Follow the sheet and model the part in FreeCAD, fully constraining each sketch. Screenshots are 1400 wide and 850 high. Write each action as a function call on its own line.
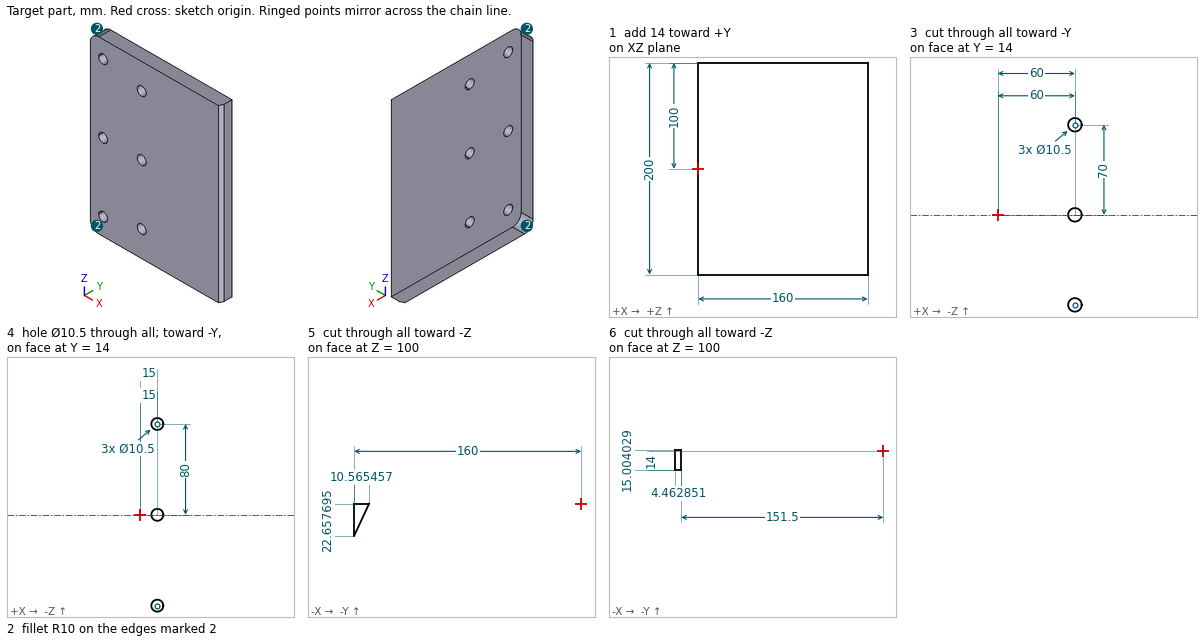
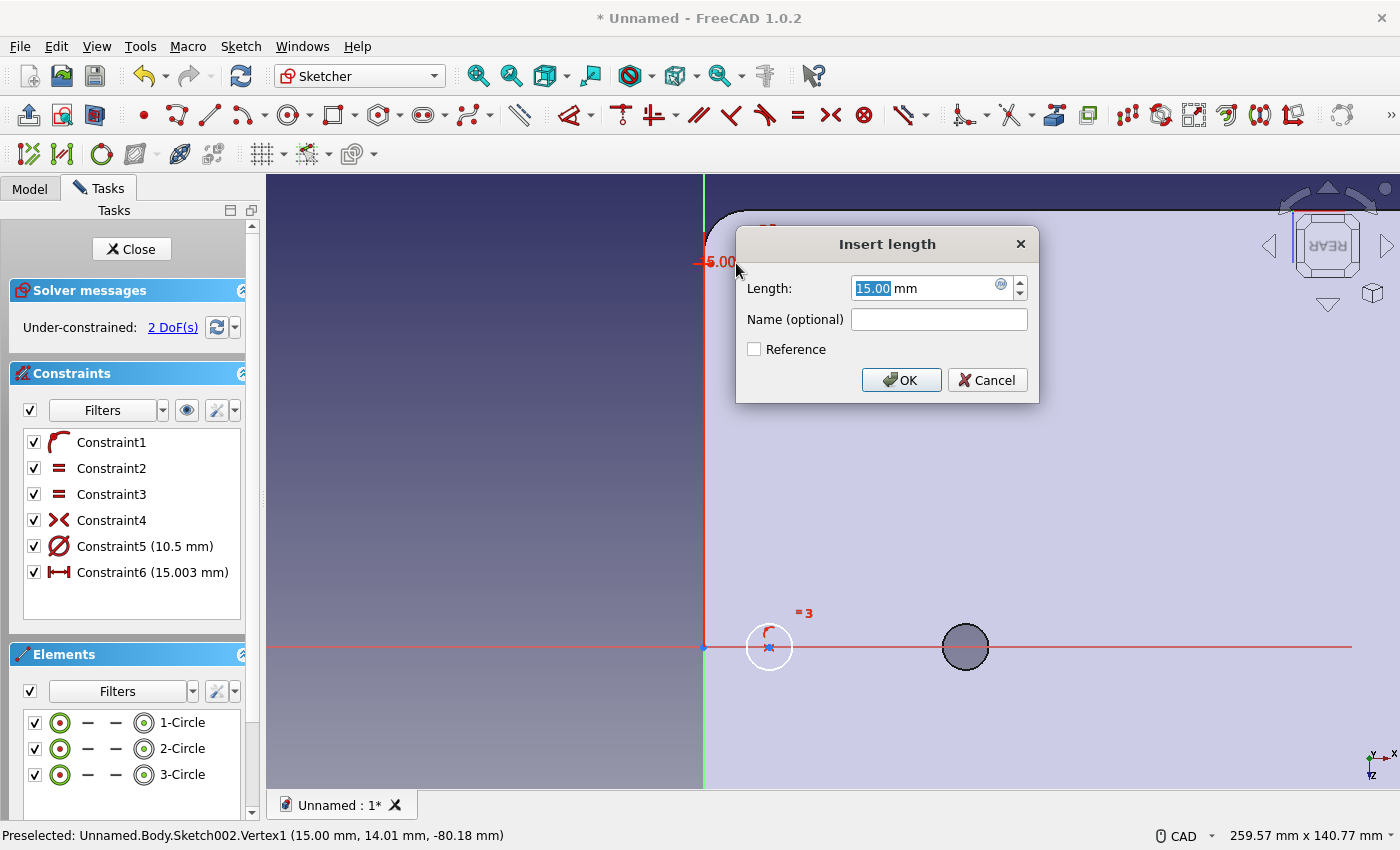
text(15)
key(Return)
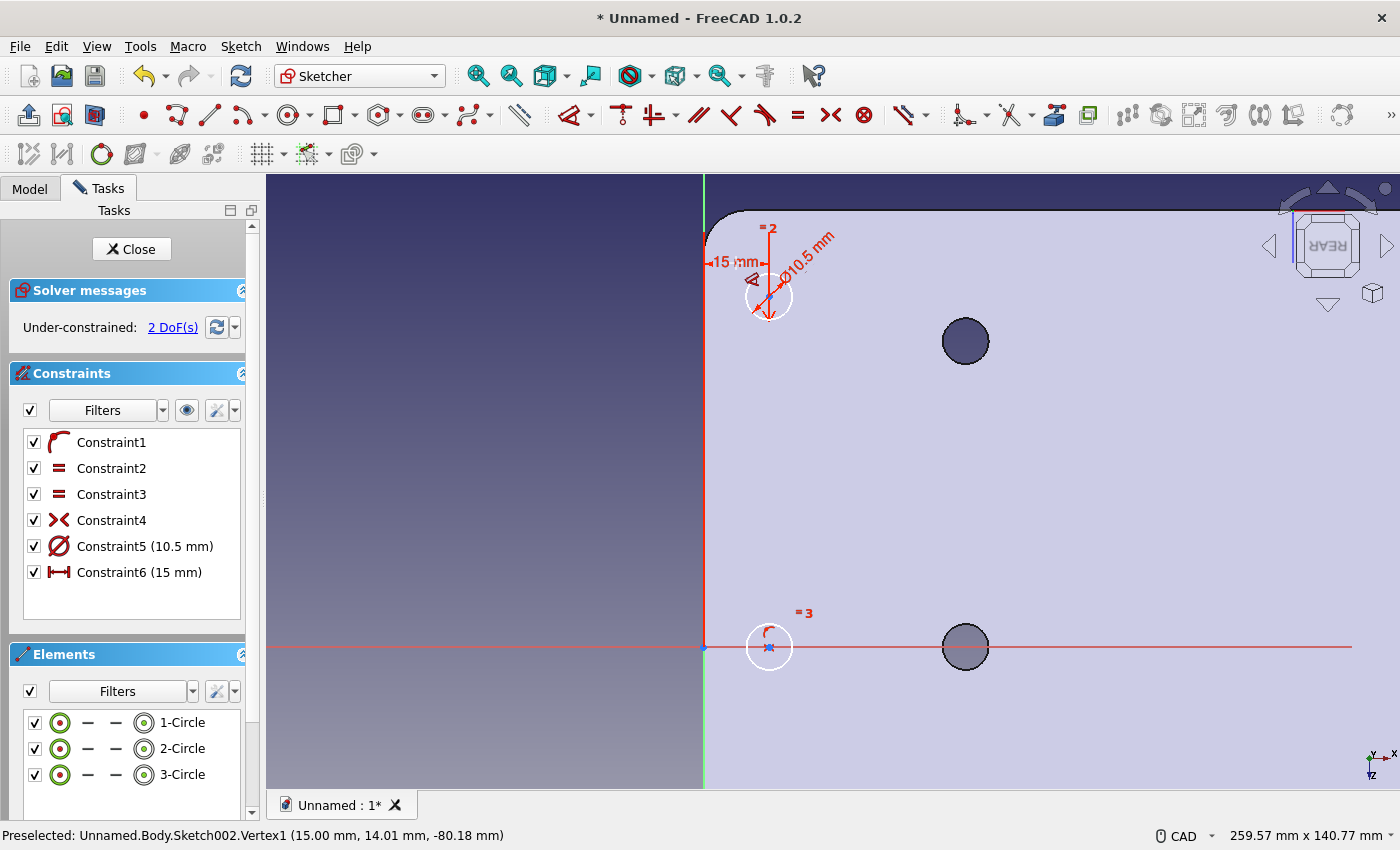
click(769, 297)
click(670, 472)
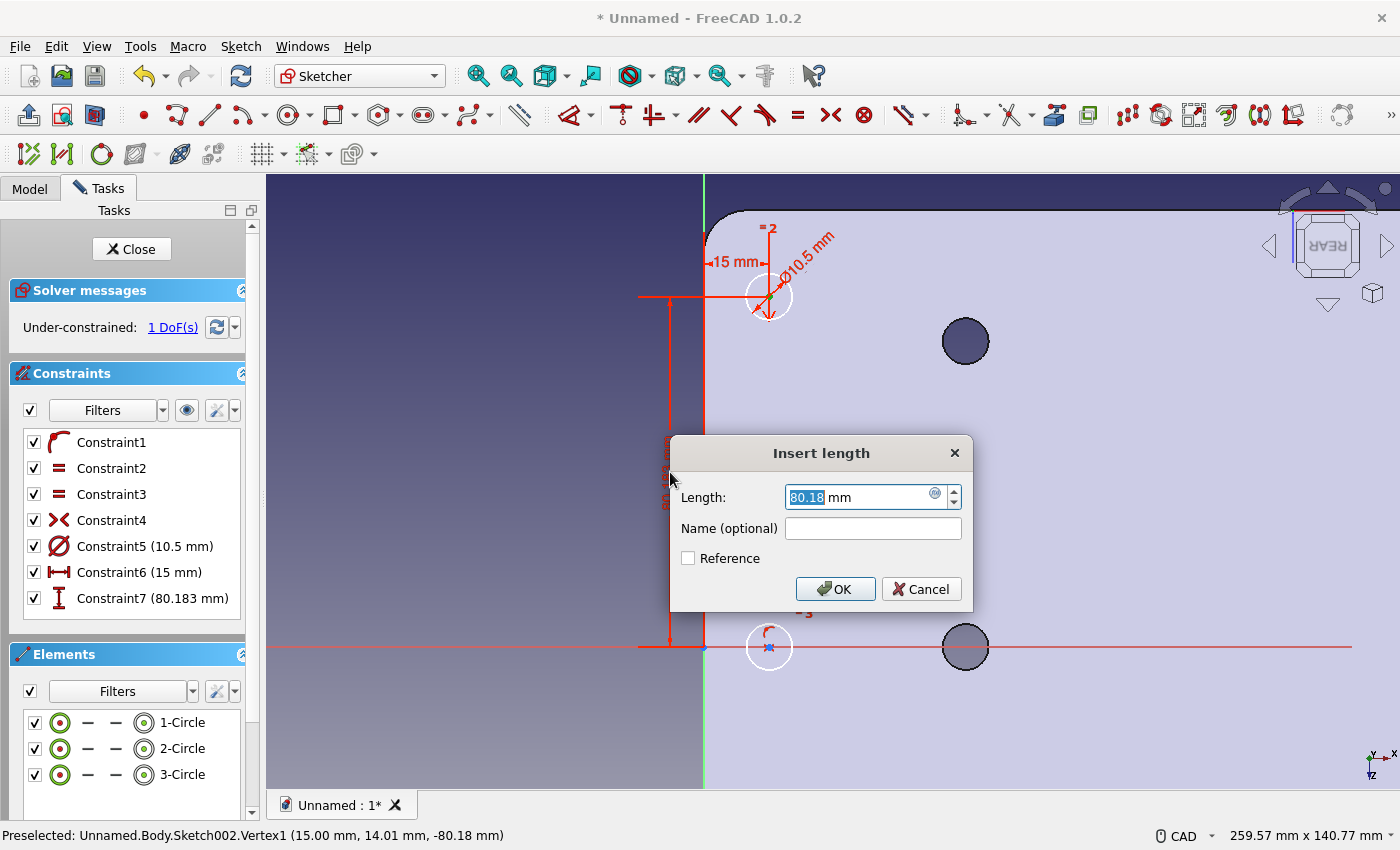
text(80)
key(Return)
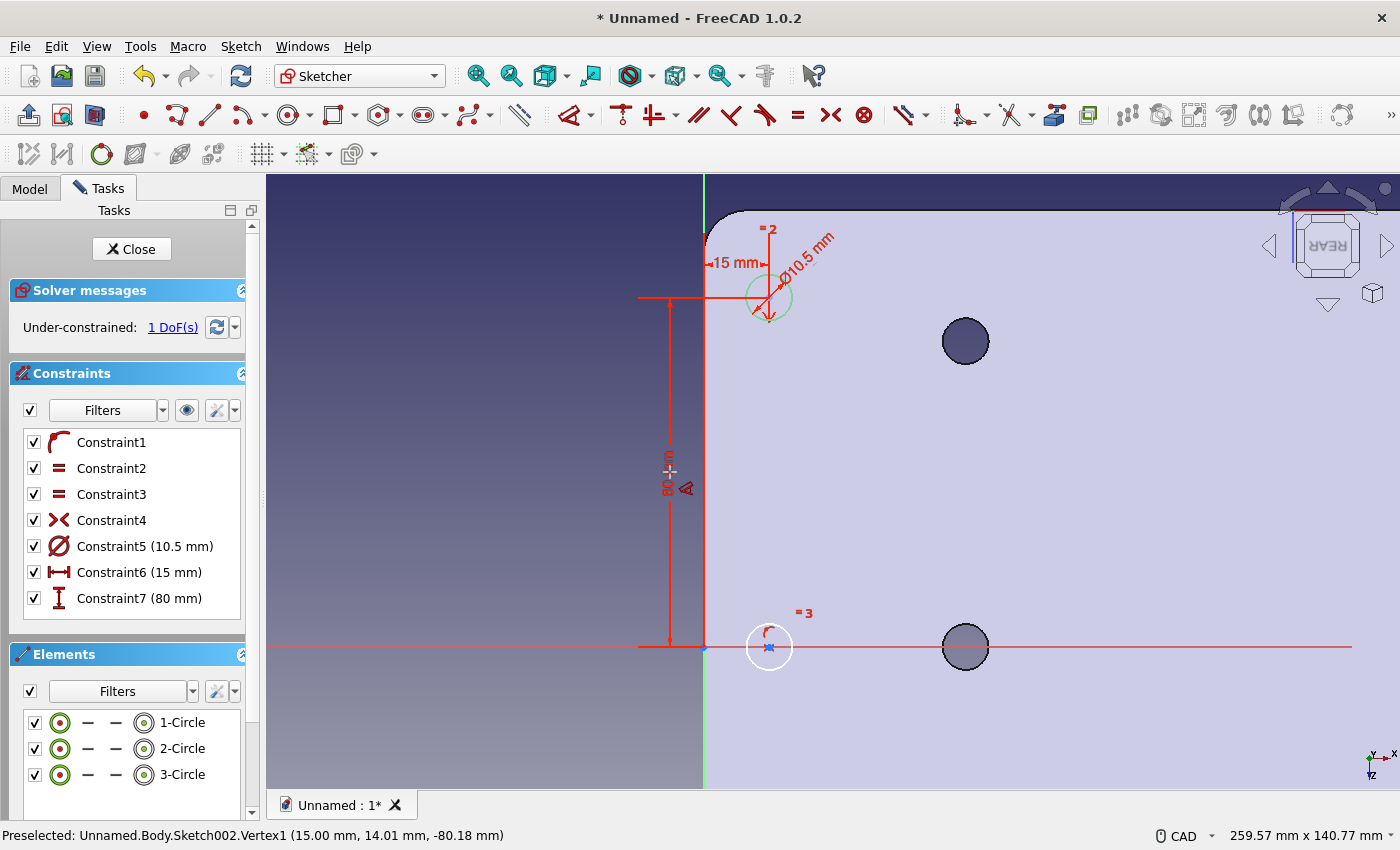
click(769, 647)
click(737, 681)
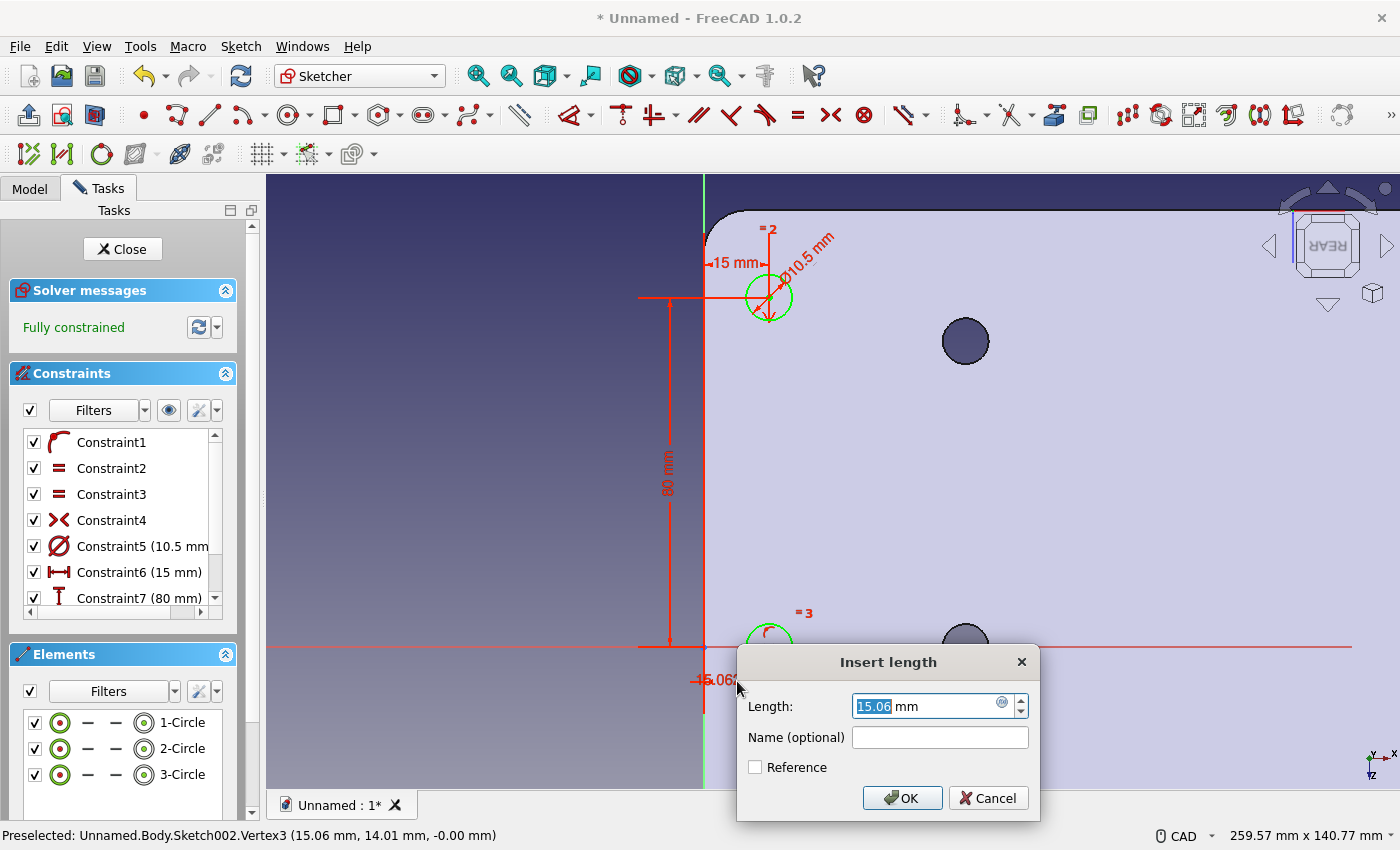
text(15)
key(Return)
key(Escape)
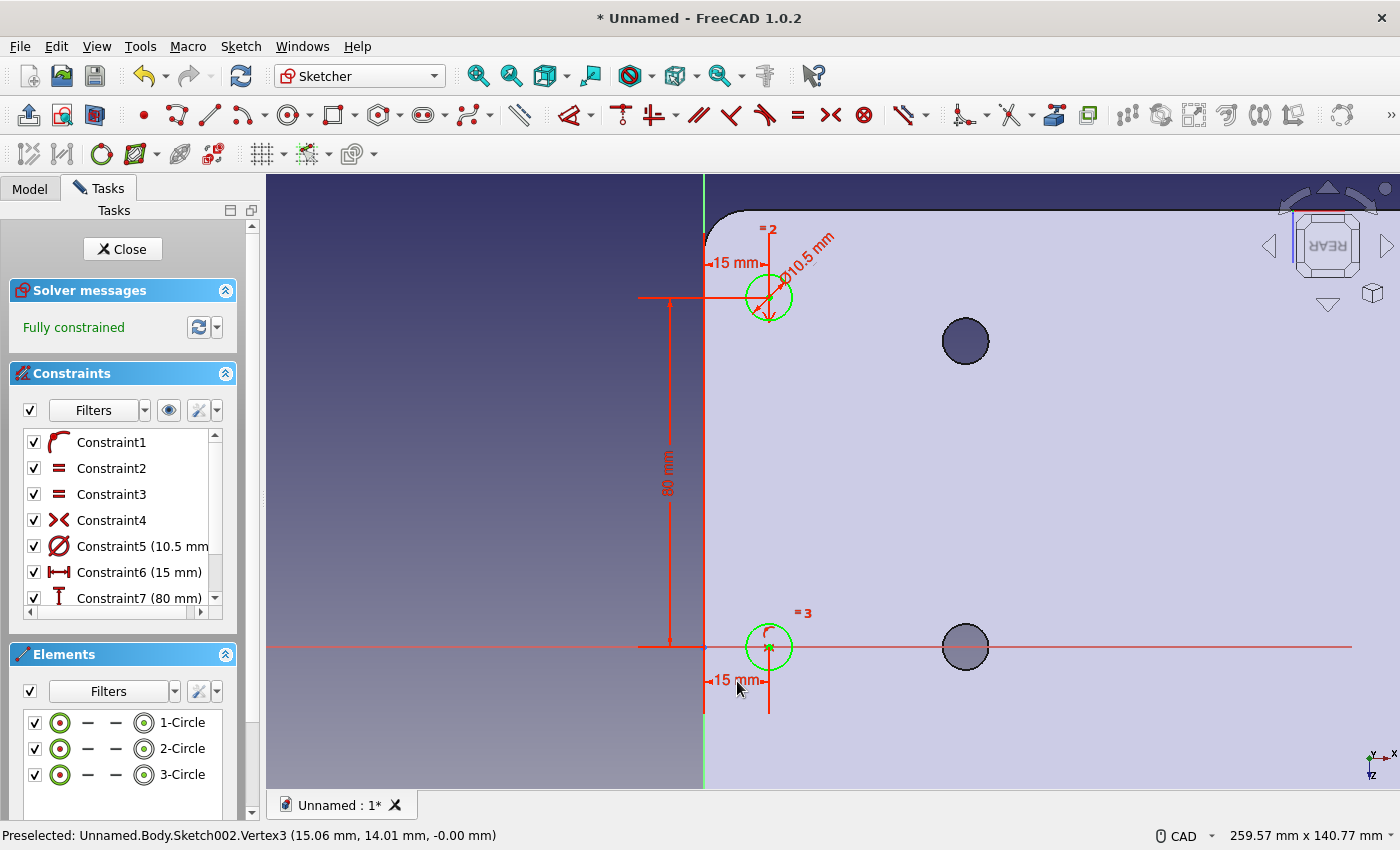
click(123, 249)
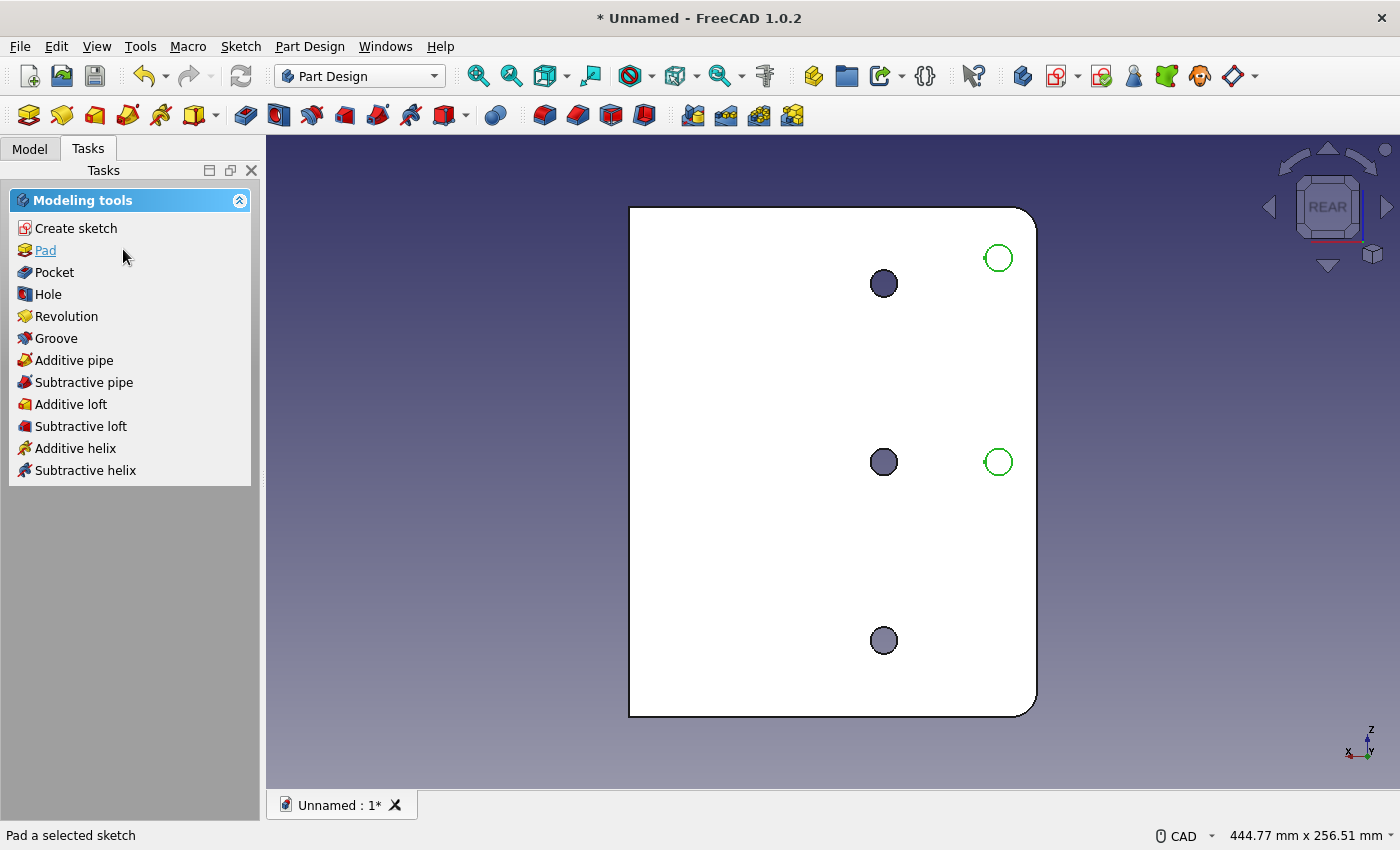
click(279, 116)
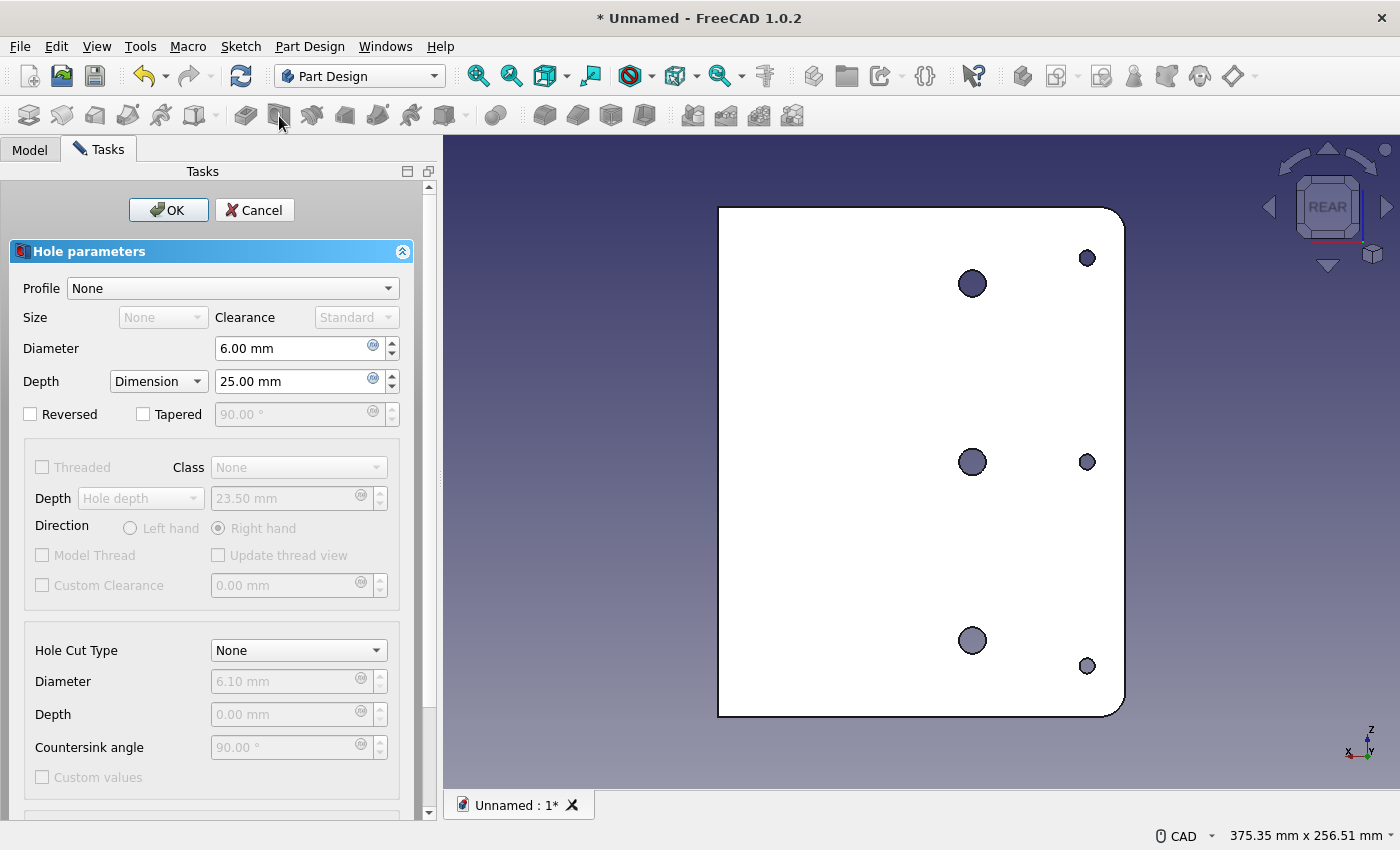
triple_click(300, 348)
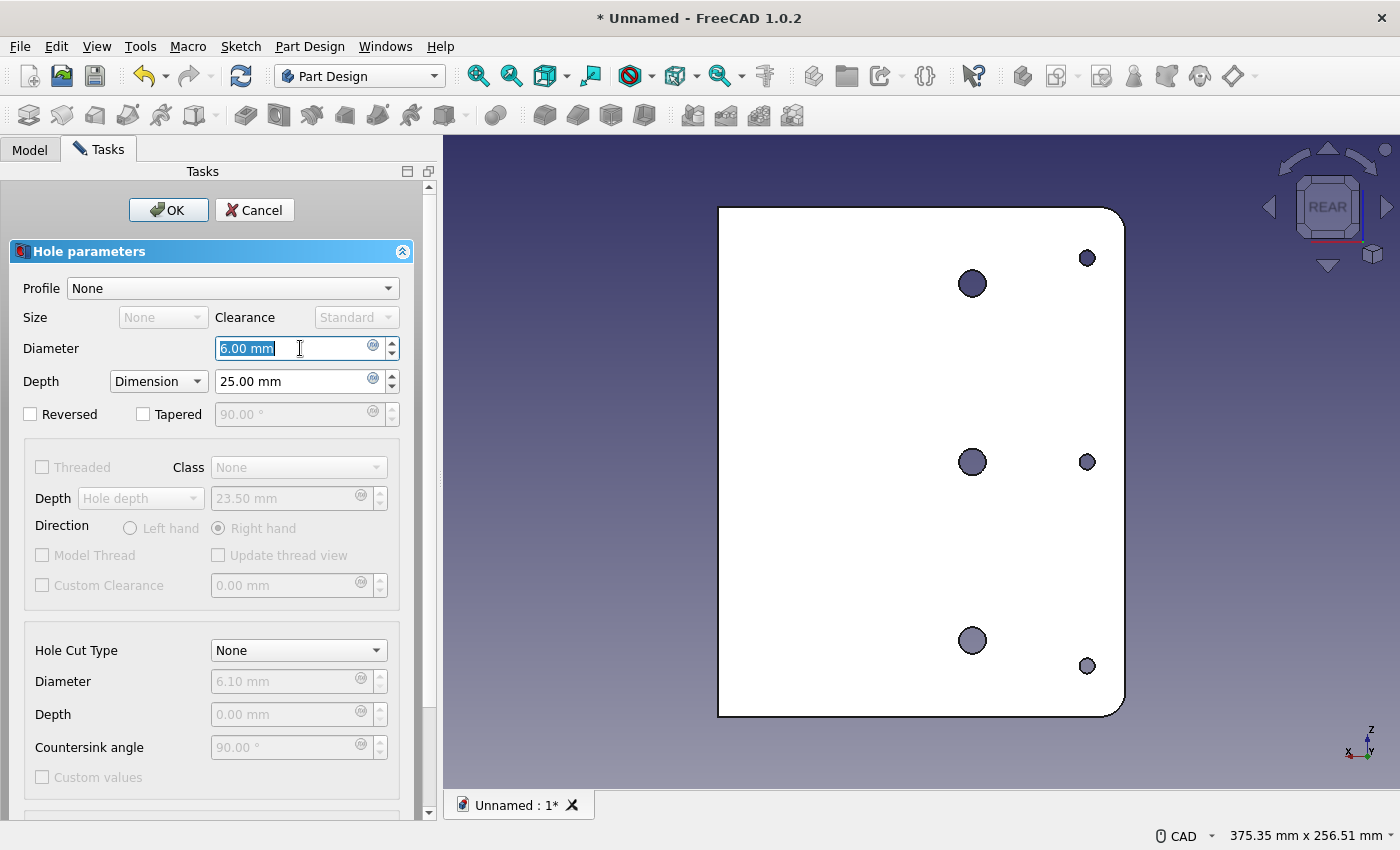
text(10.5)
key(Tab)